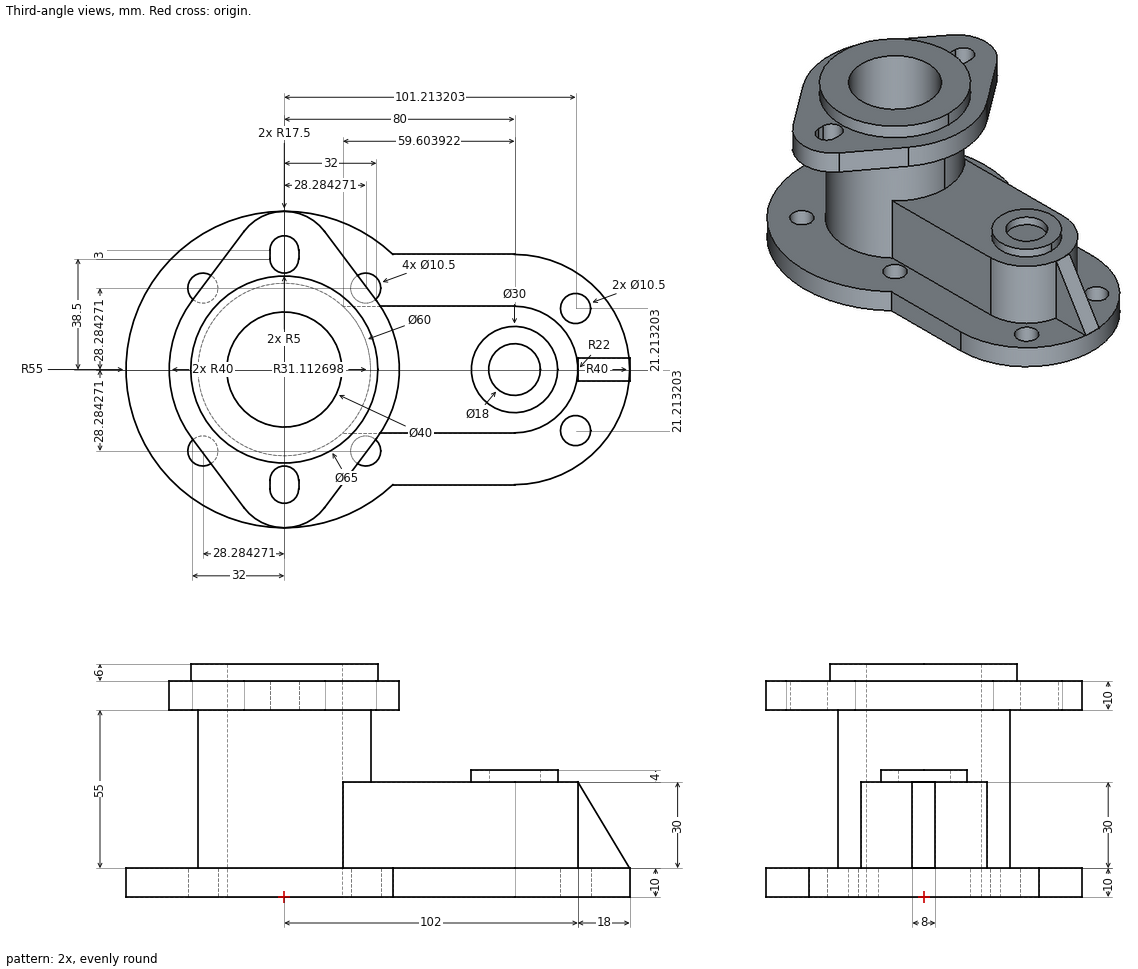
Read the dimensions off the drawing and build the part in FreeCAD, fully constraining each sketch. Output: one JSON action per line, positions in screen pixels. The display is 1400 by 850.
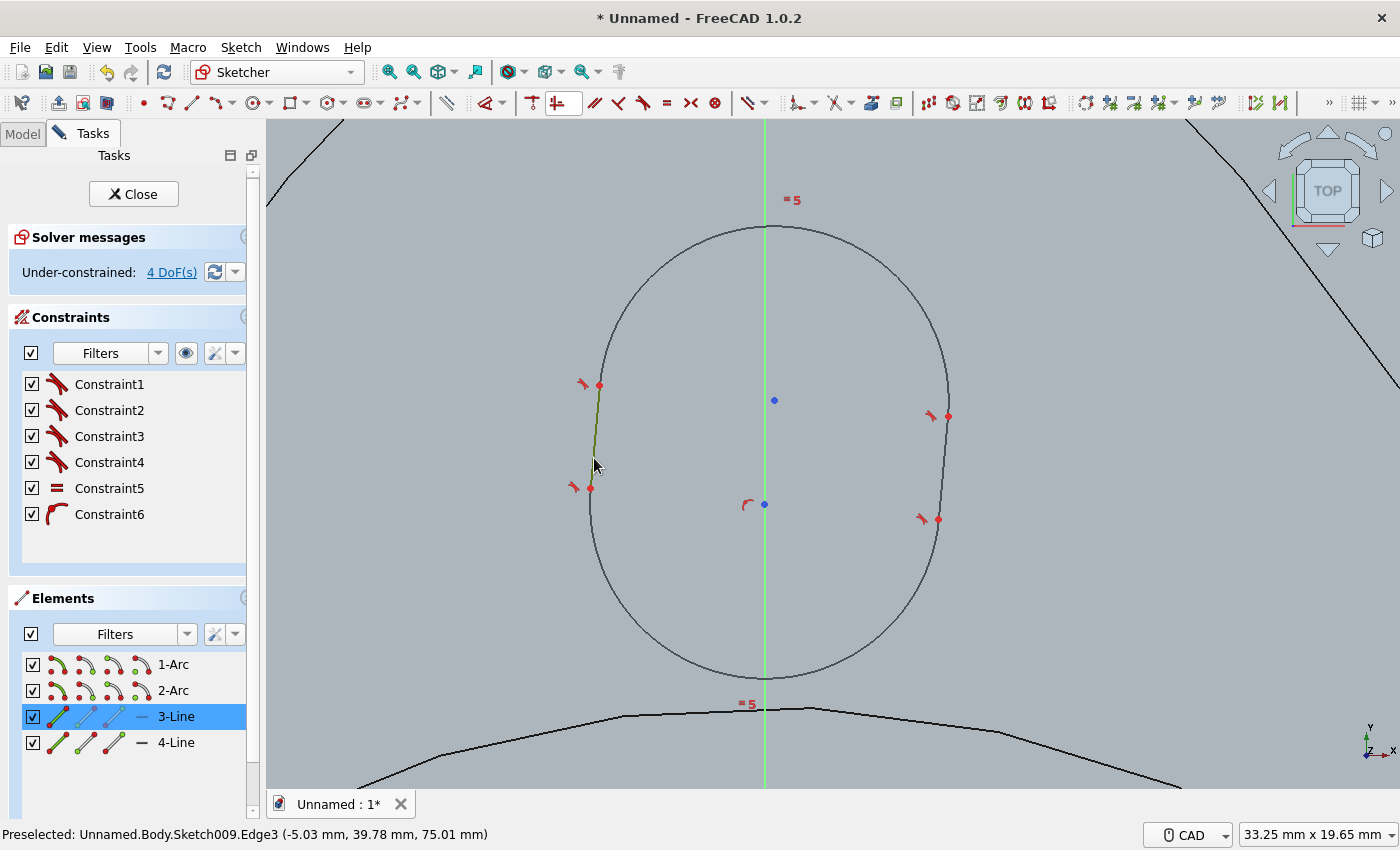
{"action": "key", "text": "v"}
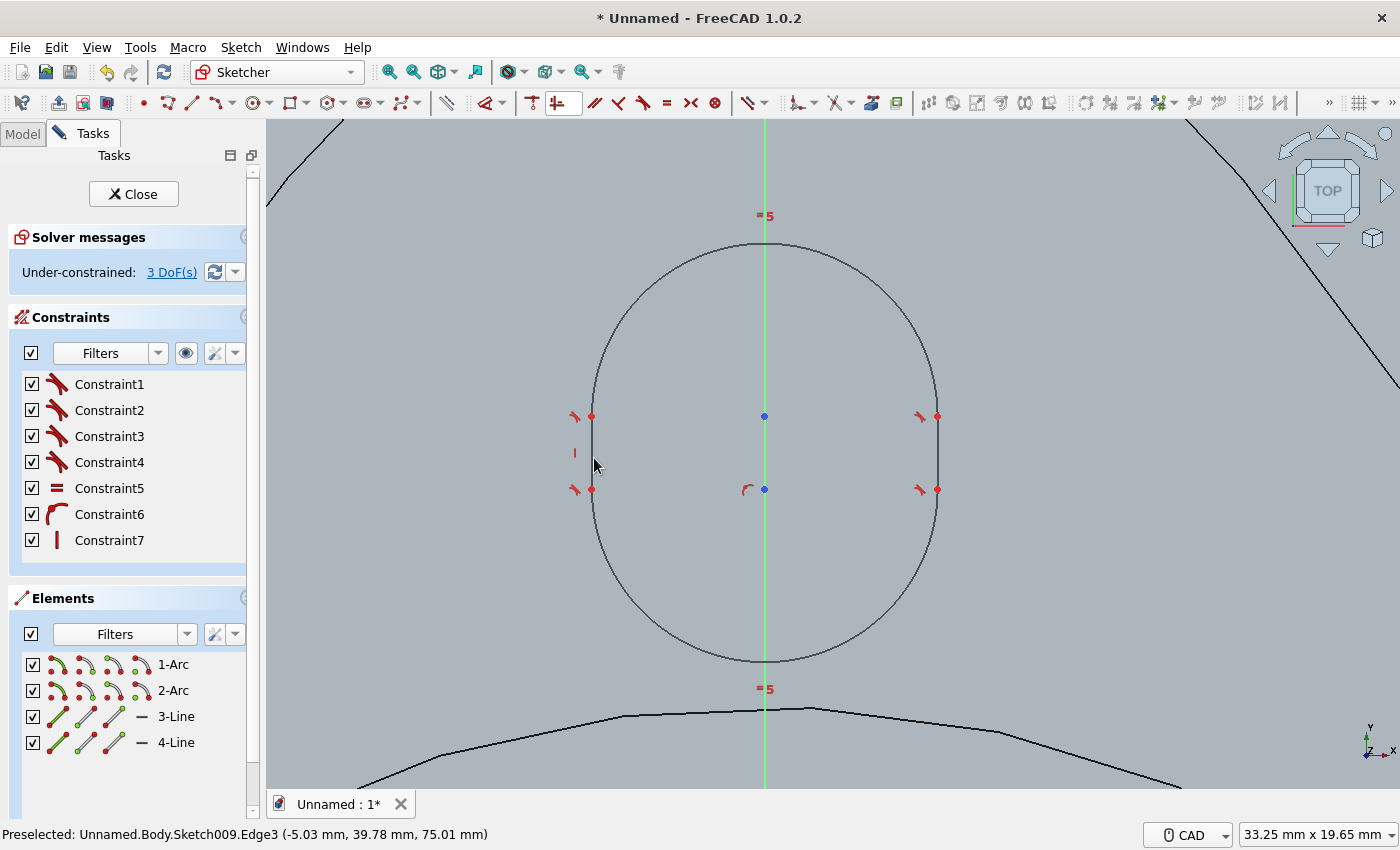
{"action": "key", "text": "d"}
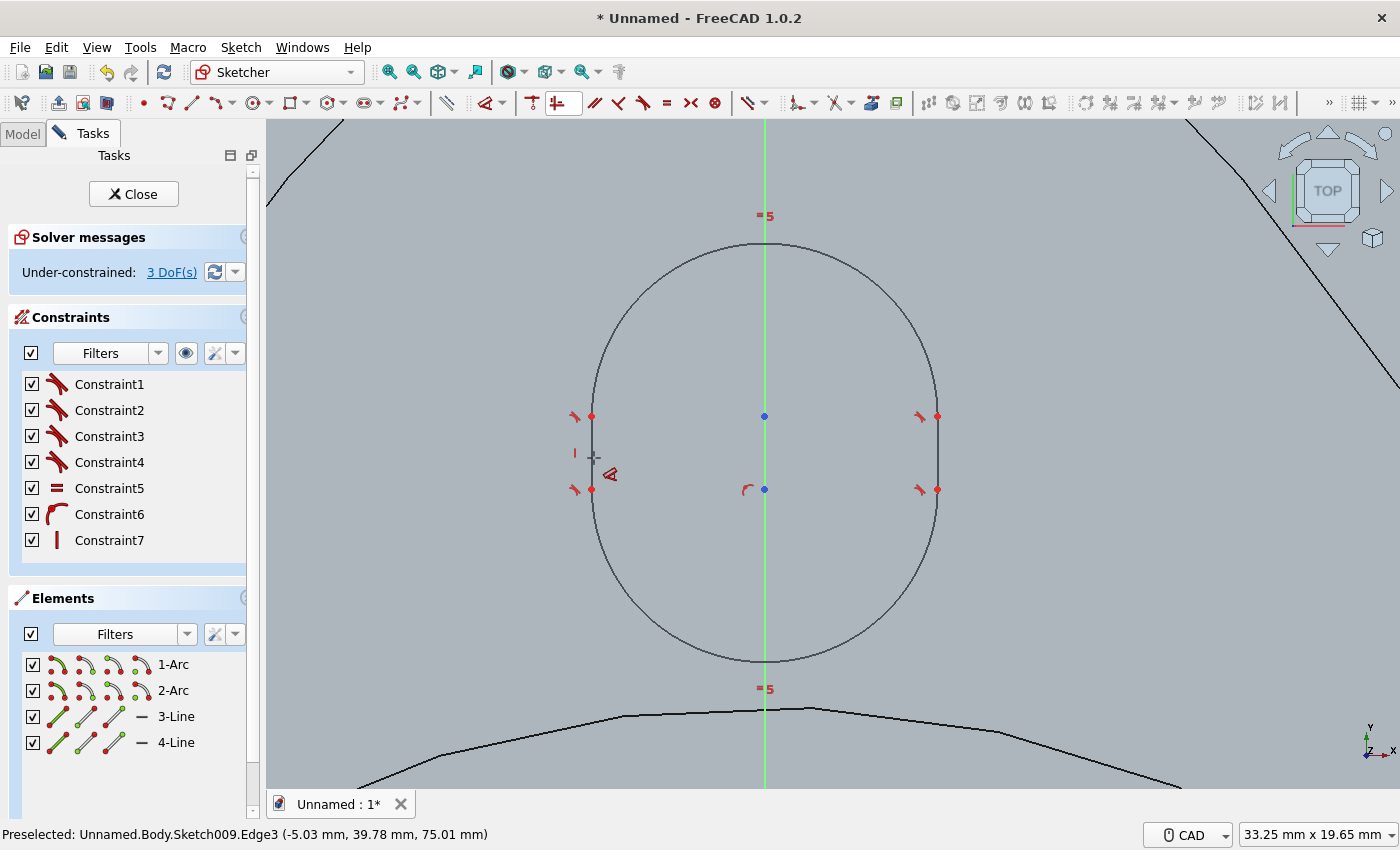
{"action": "left_click", "coordinate": [663, 629]}
{"action": "left_click", "coordinate": [644, 655]}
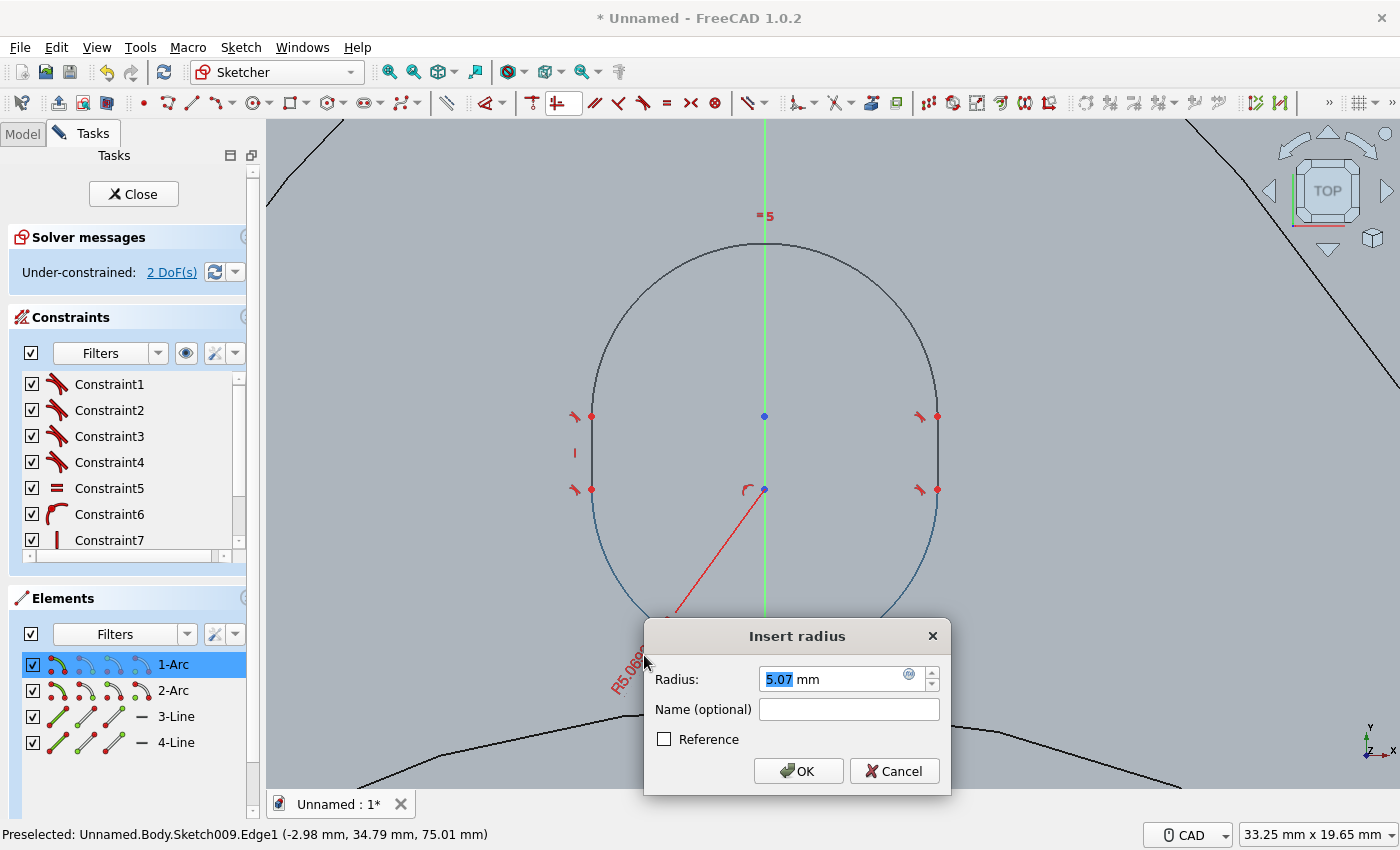
{"action": "type", "text": "5"}
{"action": "key", "text": "Return"}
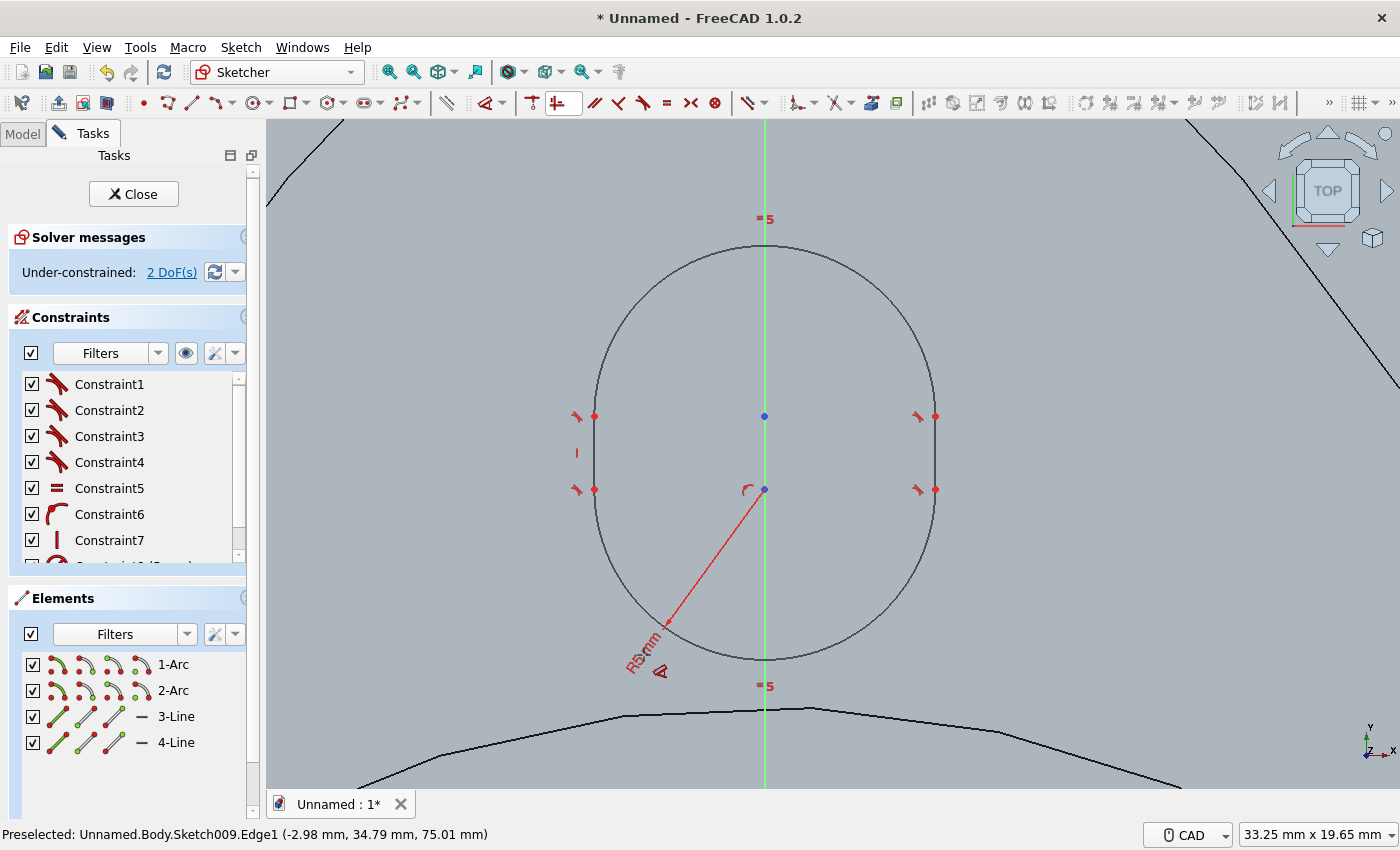
{"action": "left_click", "coordinate": [594, 467]}
{"action": "left_click", "coordinate": [560, 453]}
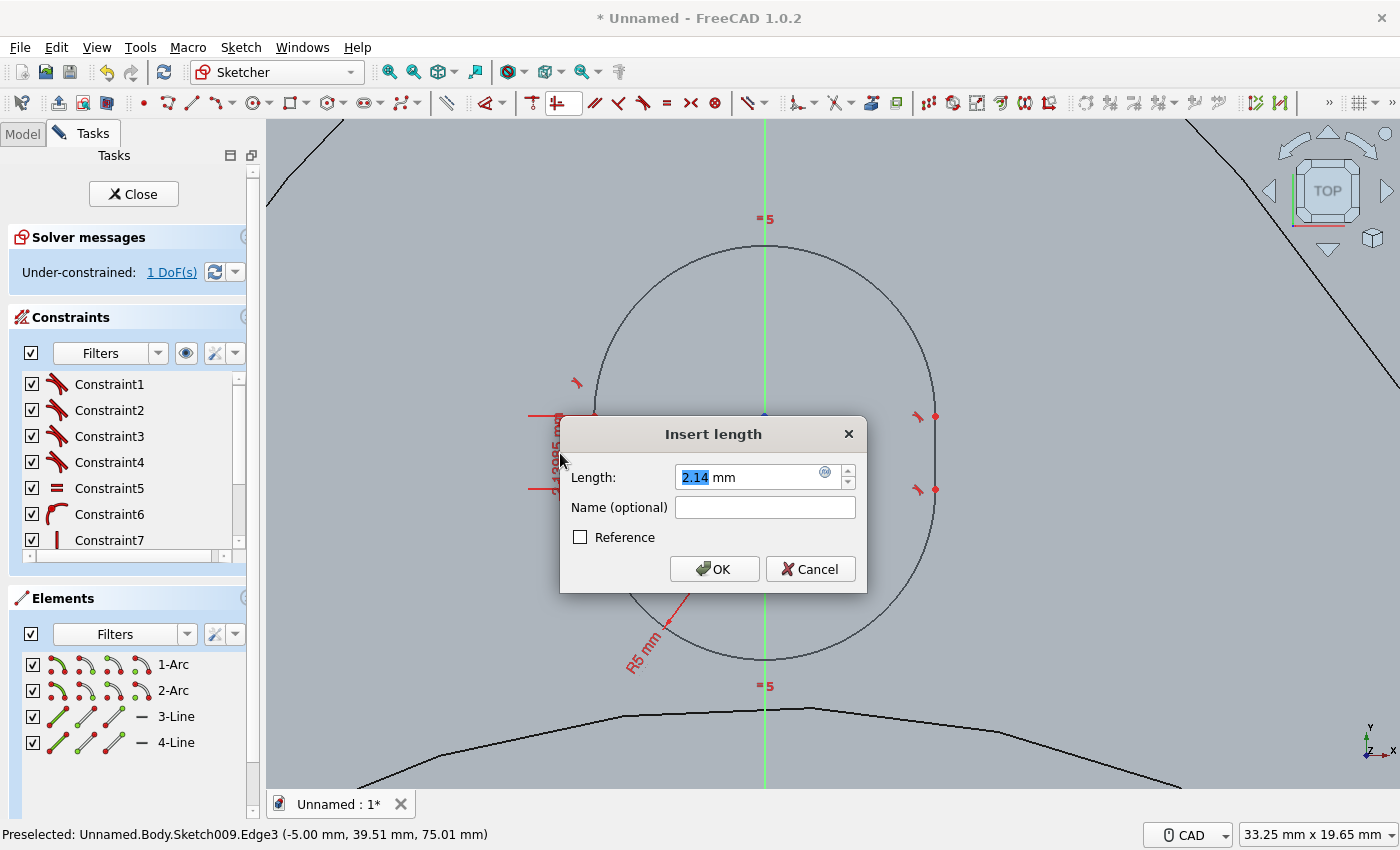
{"action": "type", "text": "3"}
{"action": "key", "text": "Return"}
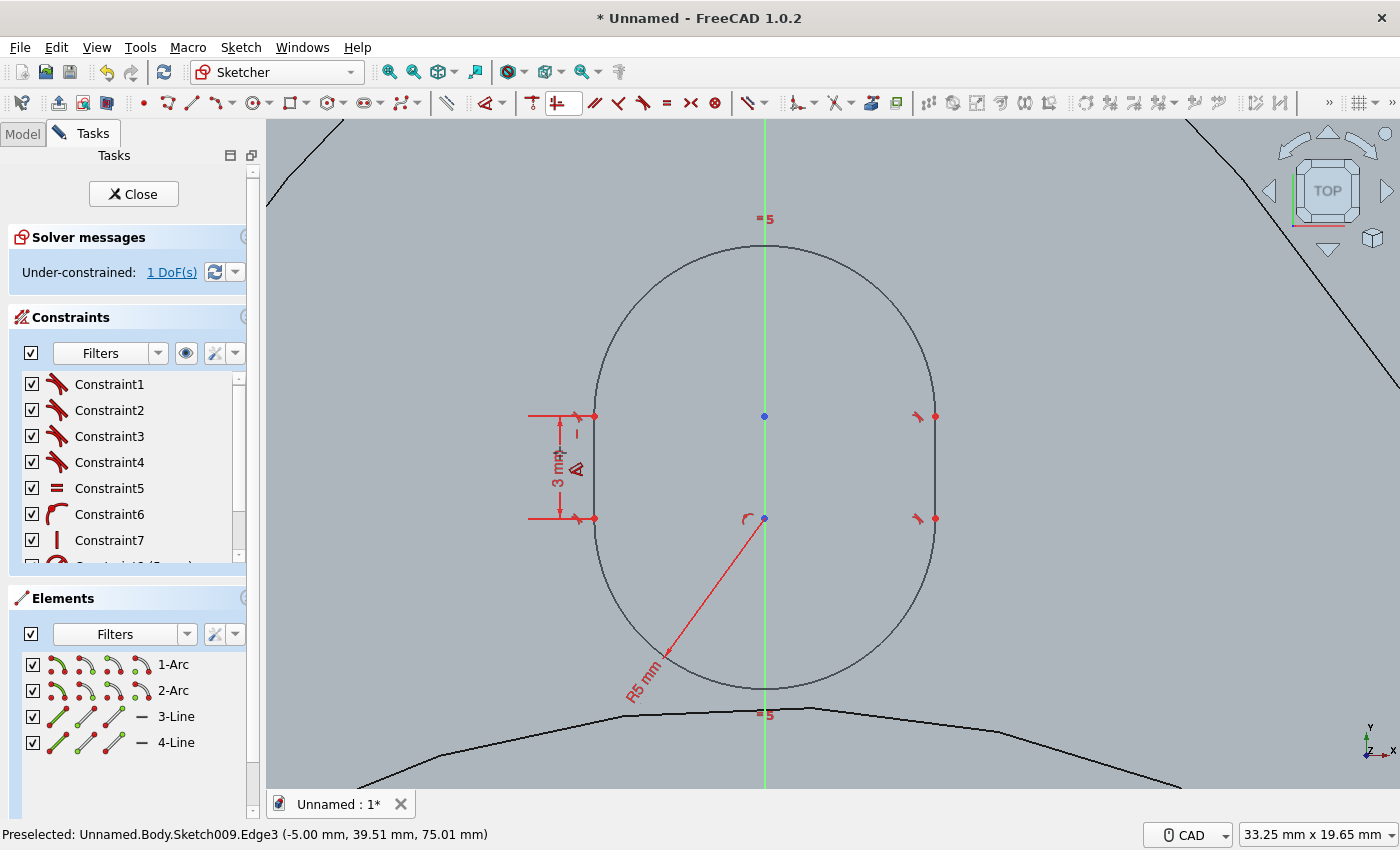
{"action": "left_click", "coordinate": [594, 519]}
{"action": "left_click", "coordinate": [560, 640]}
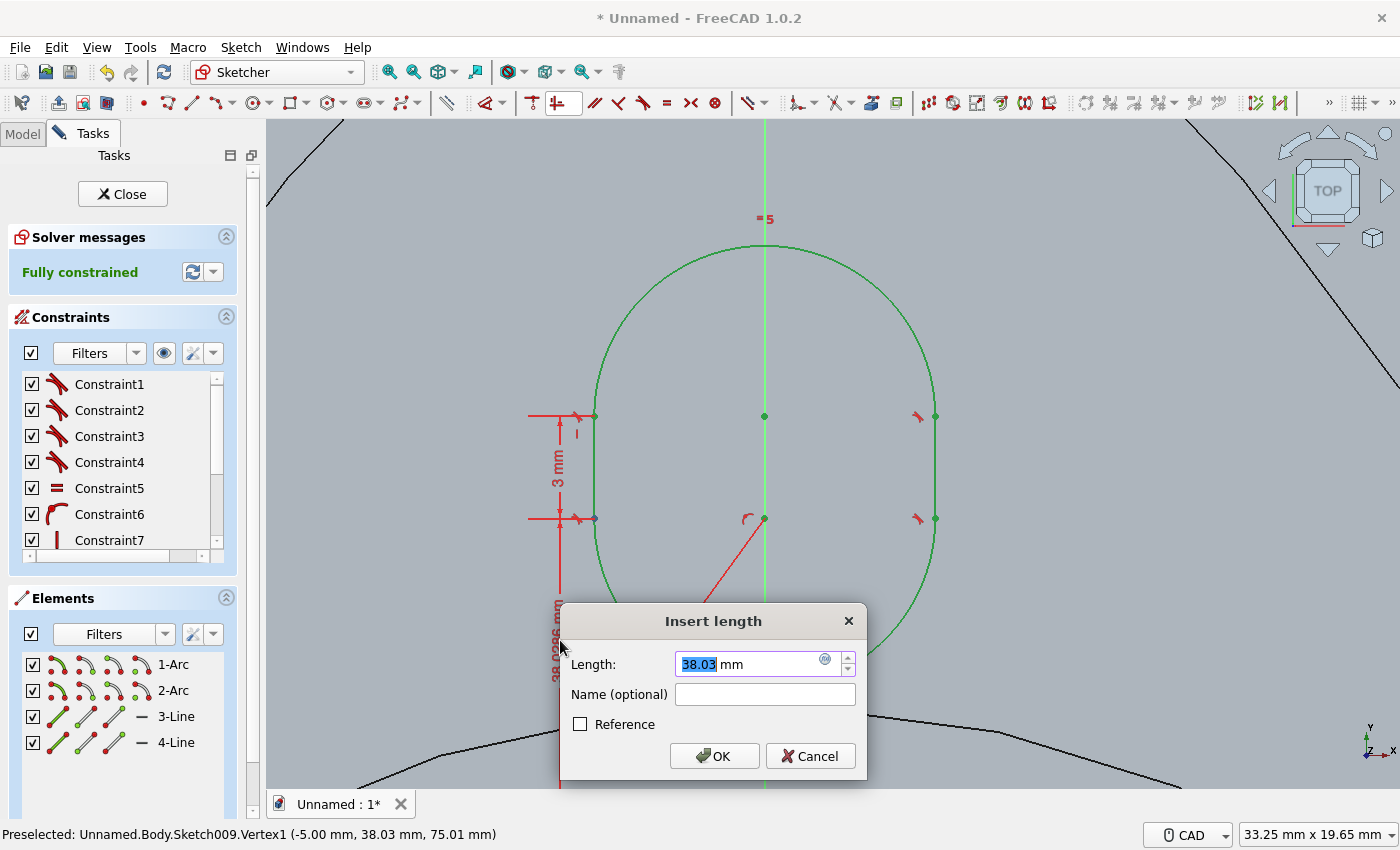
{"action": "type", "text": "38.5"}
{"action": "key", "text": "Return"}
{"action": "key", "text": "Escape"}